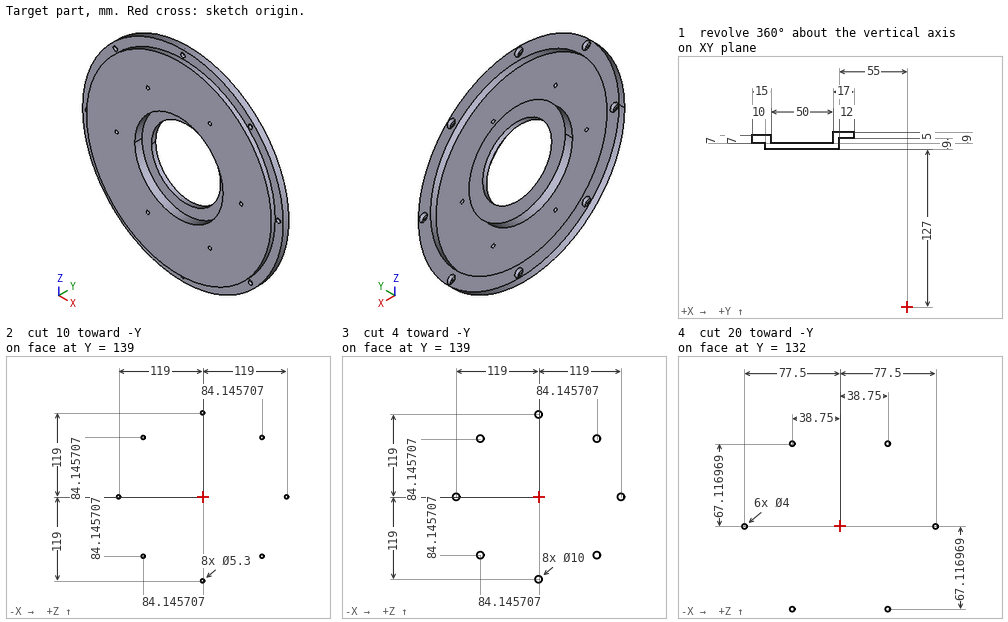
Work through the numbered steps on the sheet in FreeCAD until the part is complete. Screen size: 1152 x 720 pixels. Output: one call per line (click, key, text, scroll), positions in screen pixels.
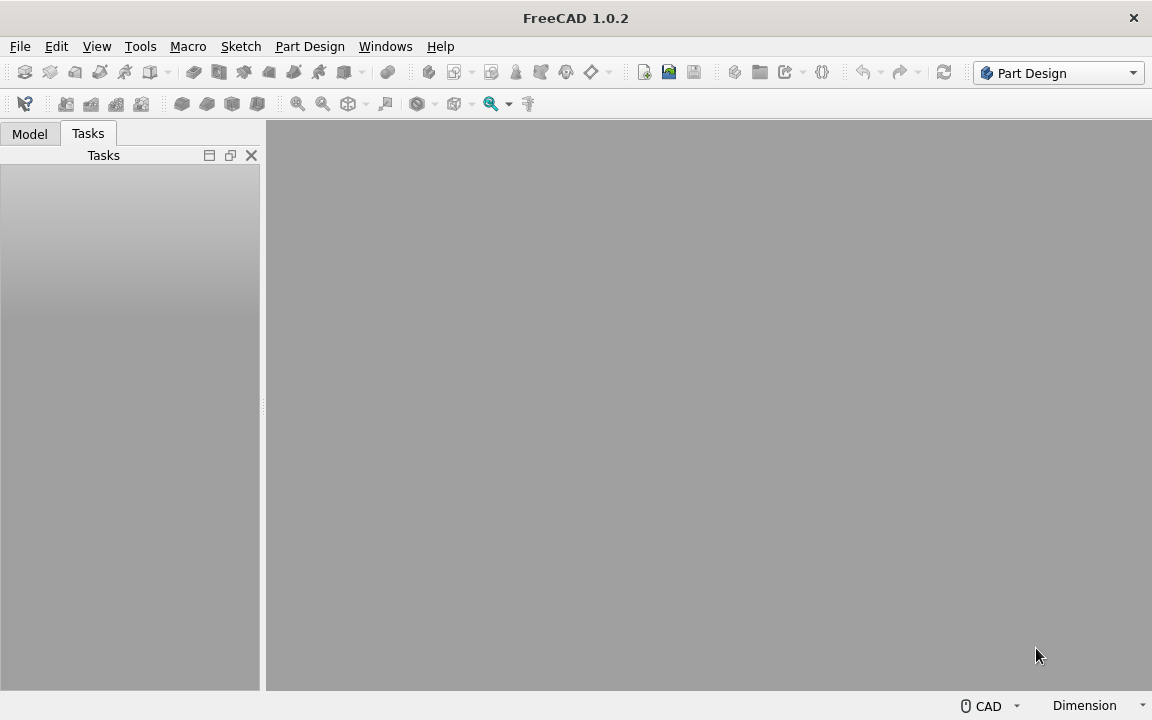
click(644, 72)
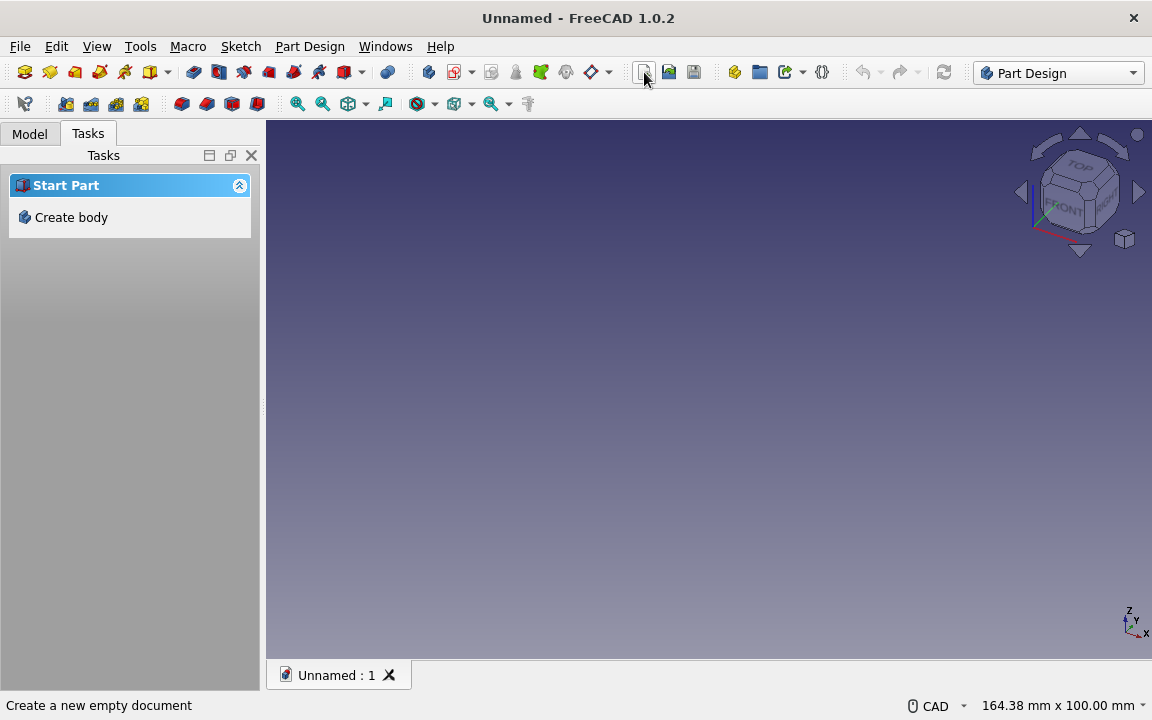
click(454, 72)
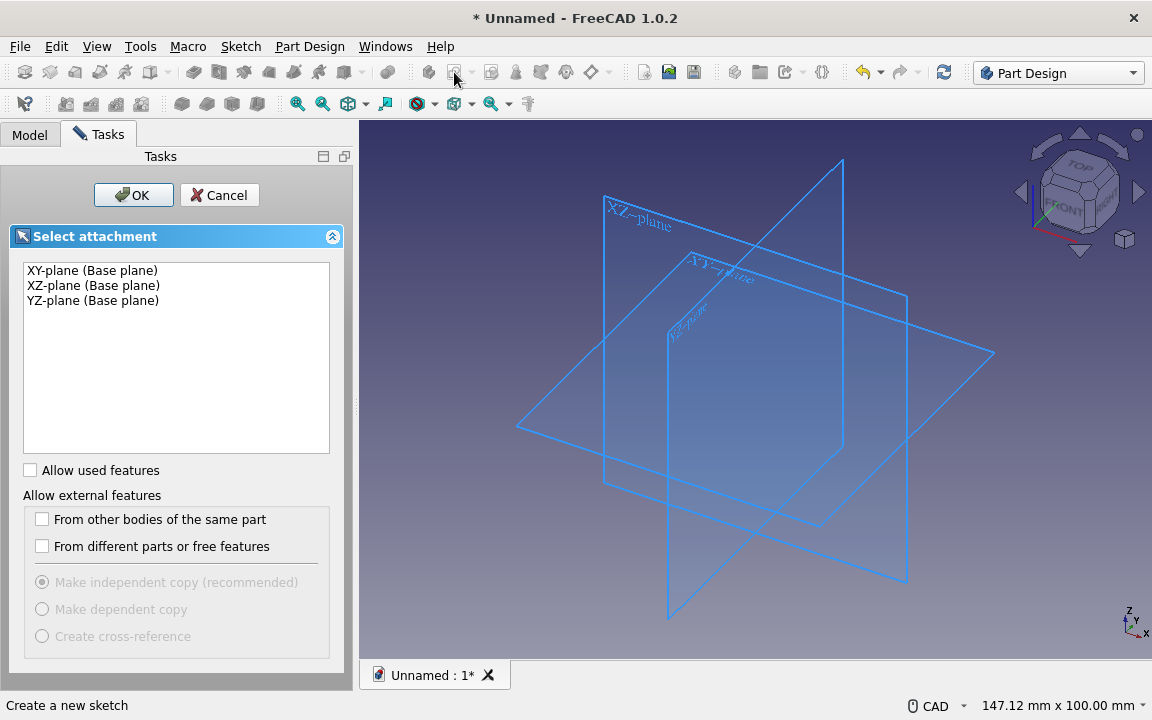
click(84, 270)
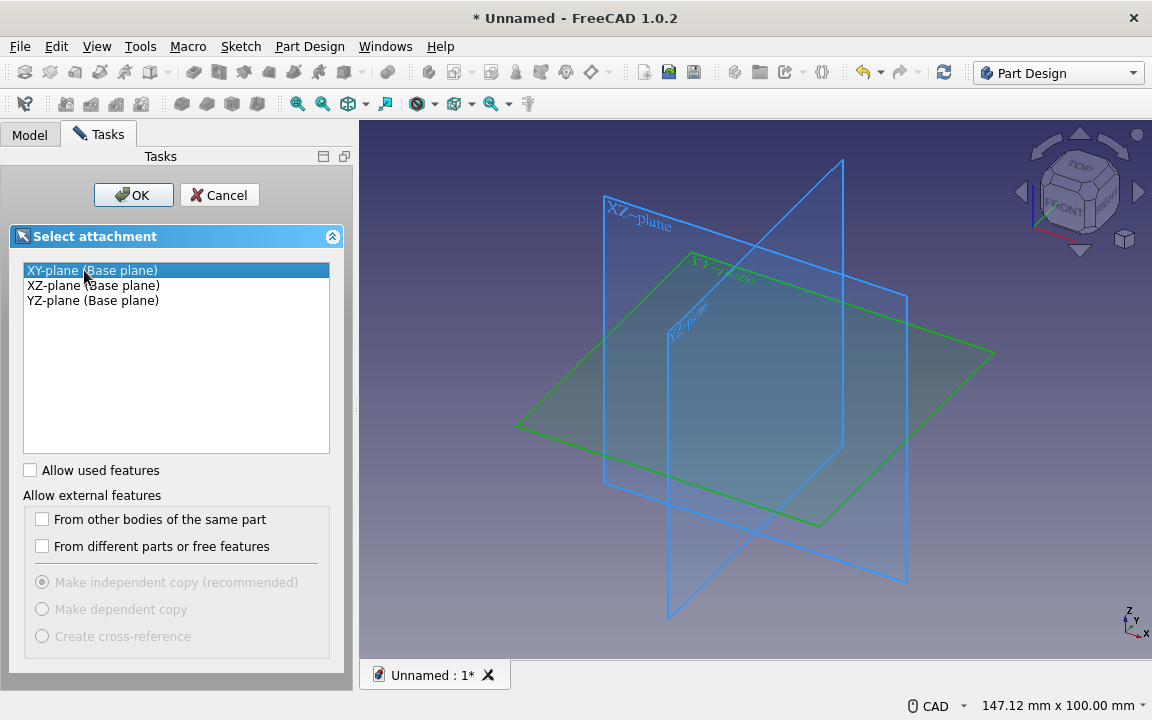
click(134, 195)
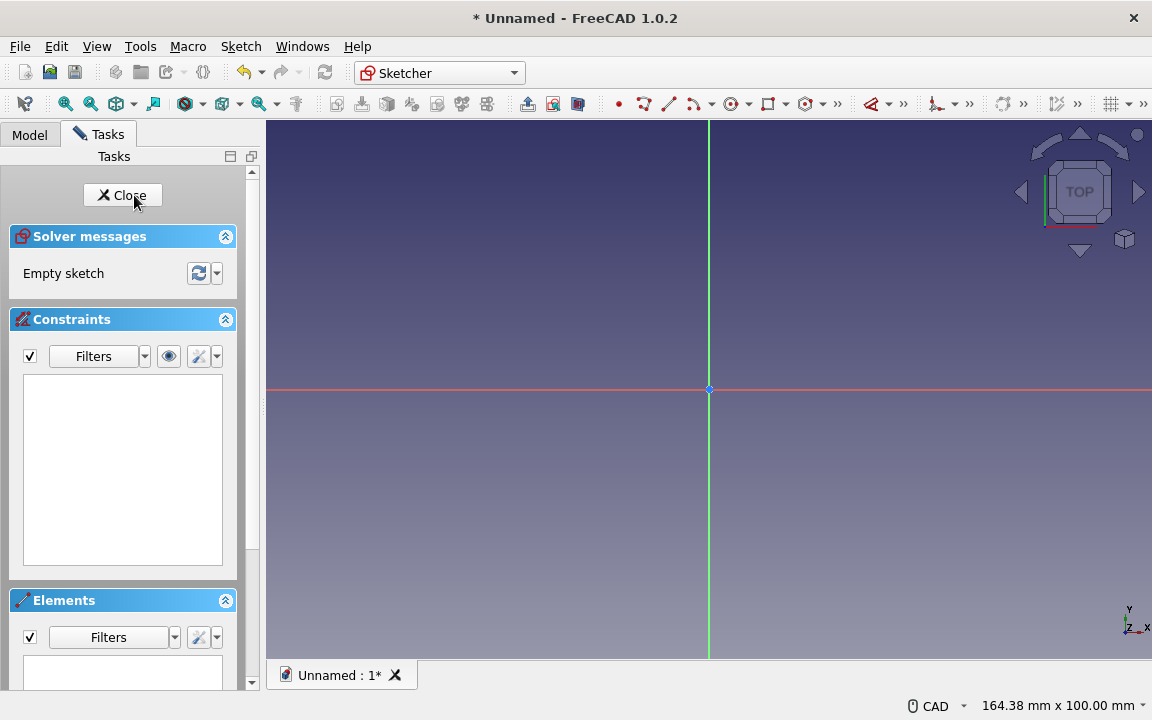
scroll(859, 631, down, 4)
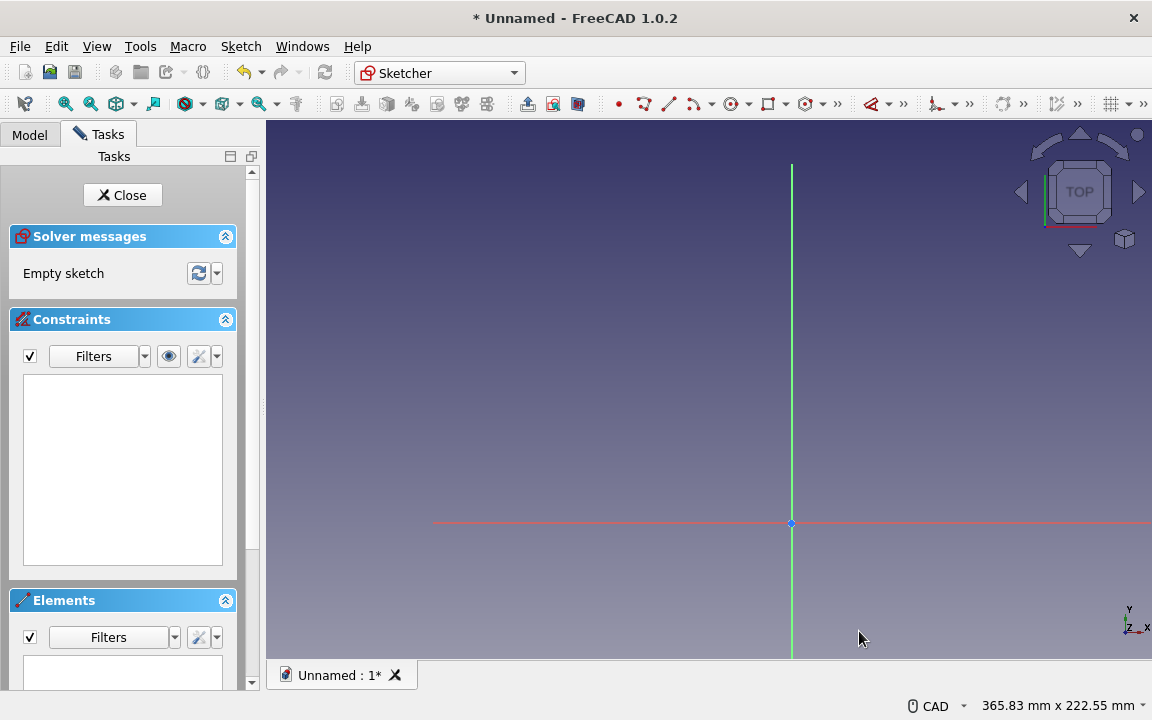
click(644, 104)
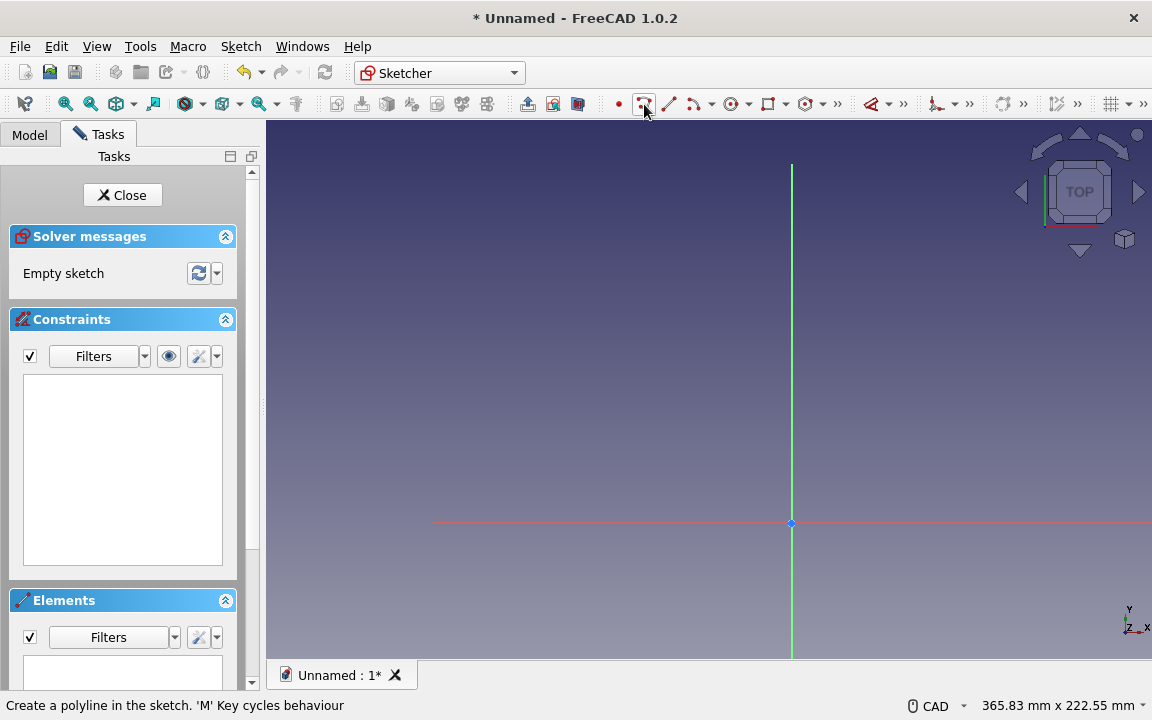
click(659, 215)
click(659, 194)
click(688, 194)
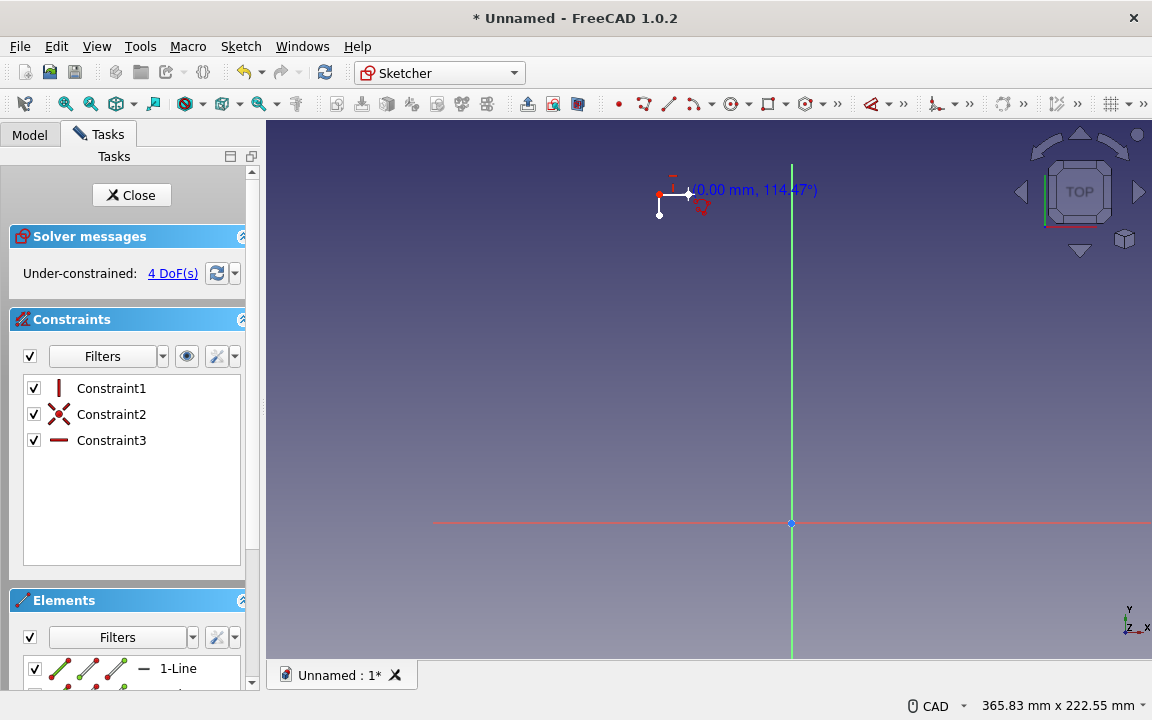
scroll(688, 182, up, 2)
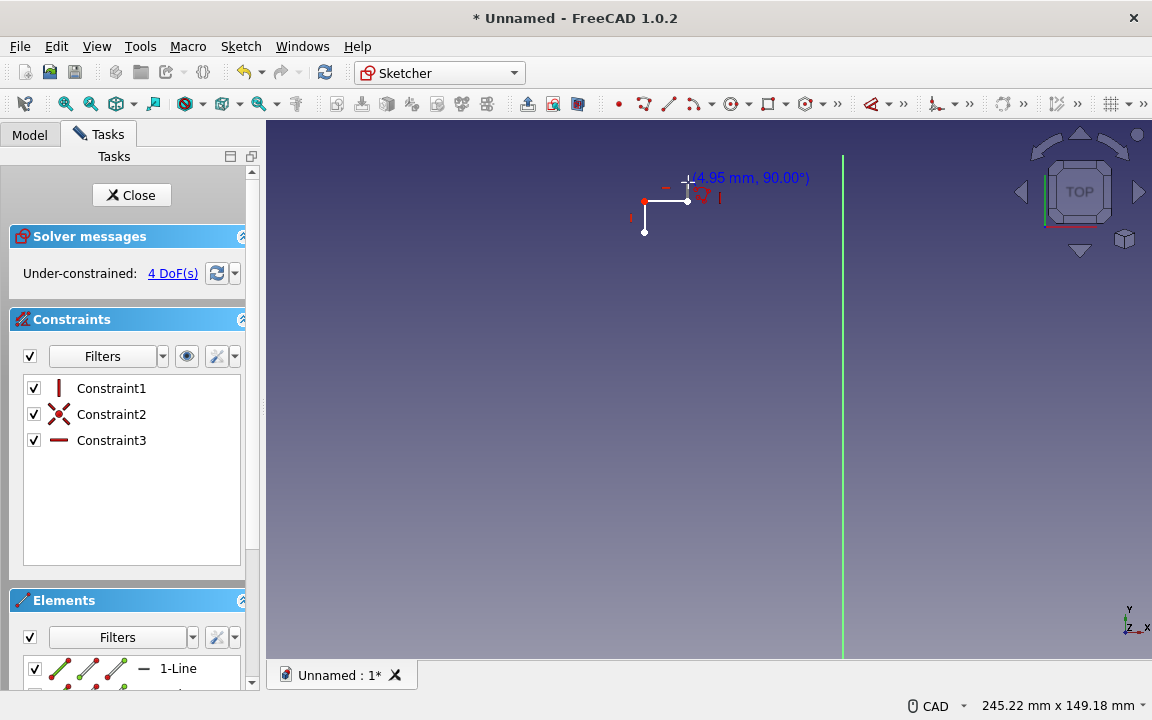
click(688, 181)
click(626, 181)
click(626, 214)
click(445, 214)
click(445, 188)
click(391, 188)
click(391, 214)
click(427, 214)
click(427, 232)
click(645, 233)
key(Escape)
key(Escape)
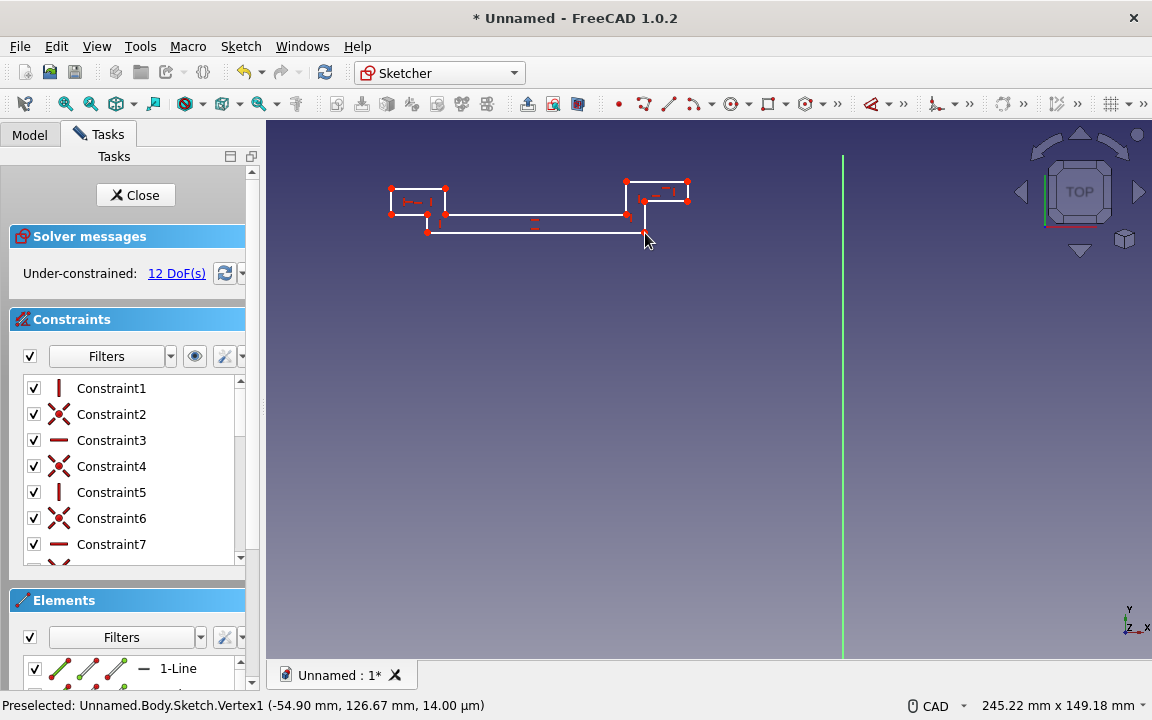
click(870, 104)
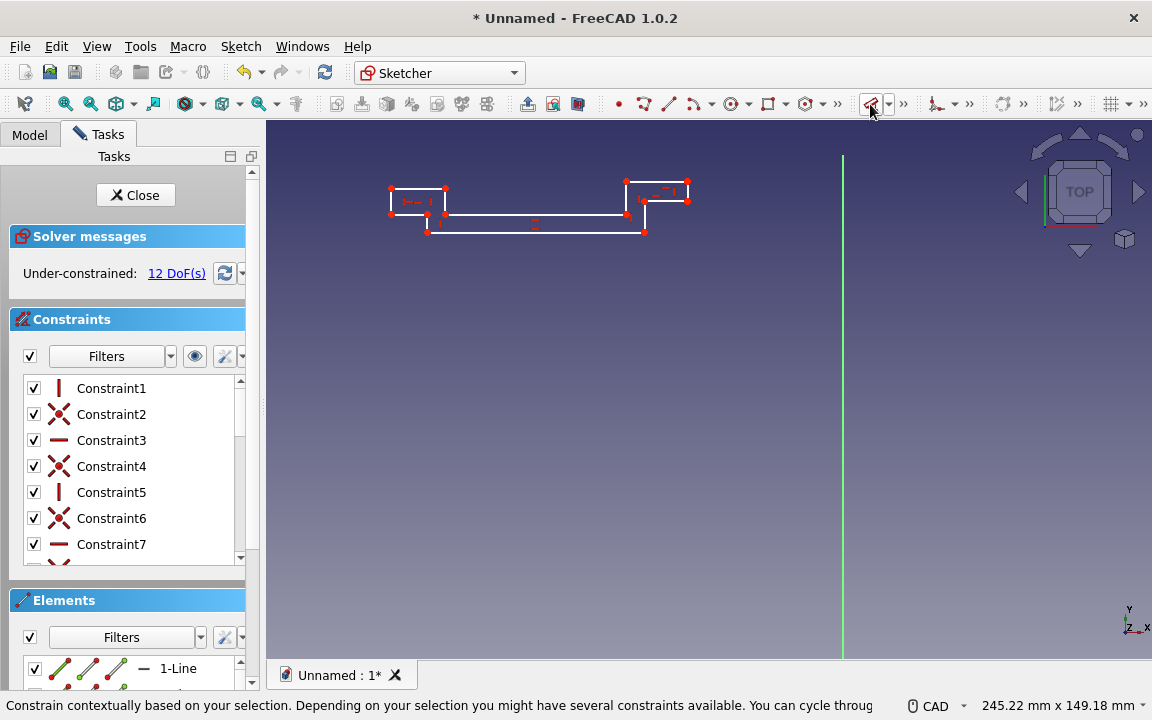
scroll(645, 224, up, 2)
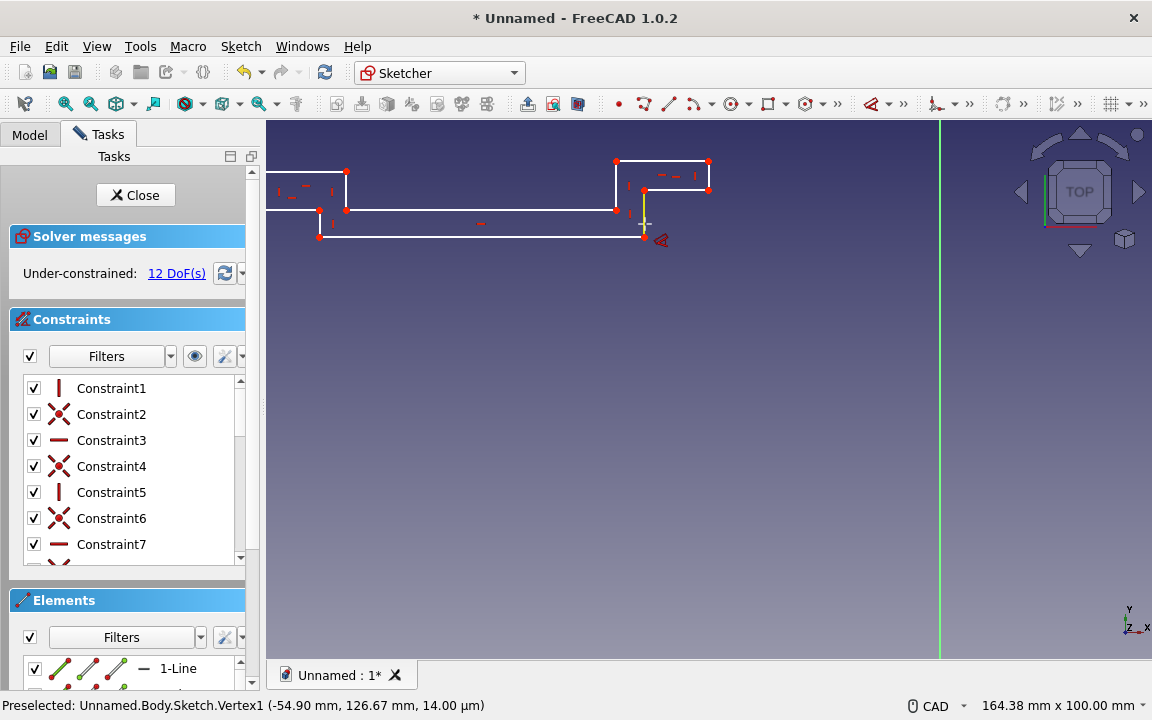
click(644, 223)
click(678, 214)